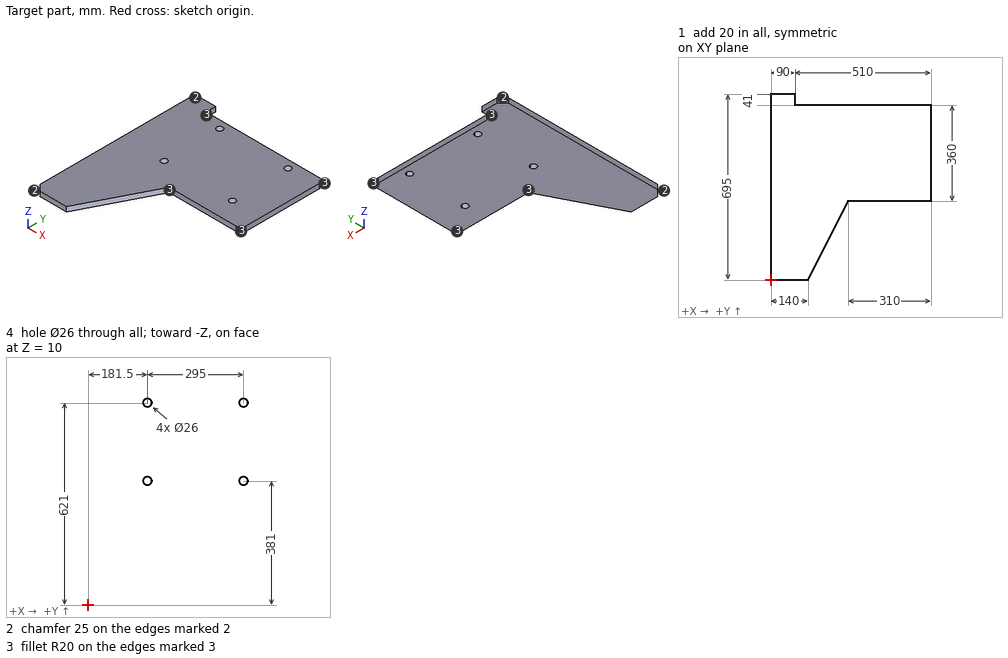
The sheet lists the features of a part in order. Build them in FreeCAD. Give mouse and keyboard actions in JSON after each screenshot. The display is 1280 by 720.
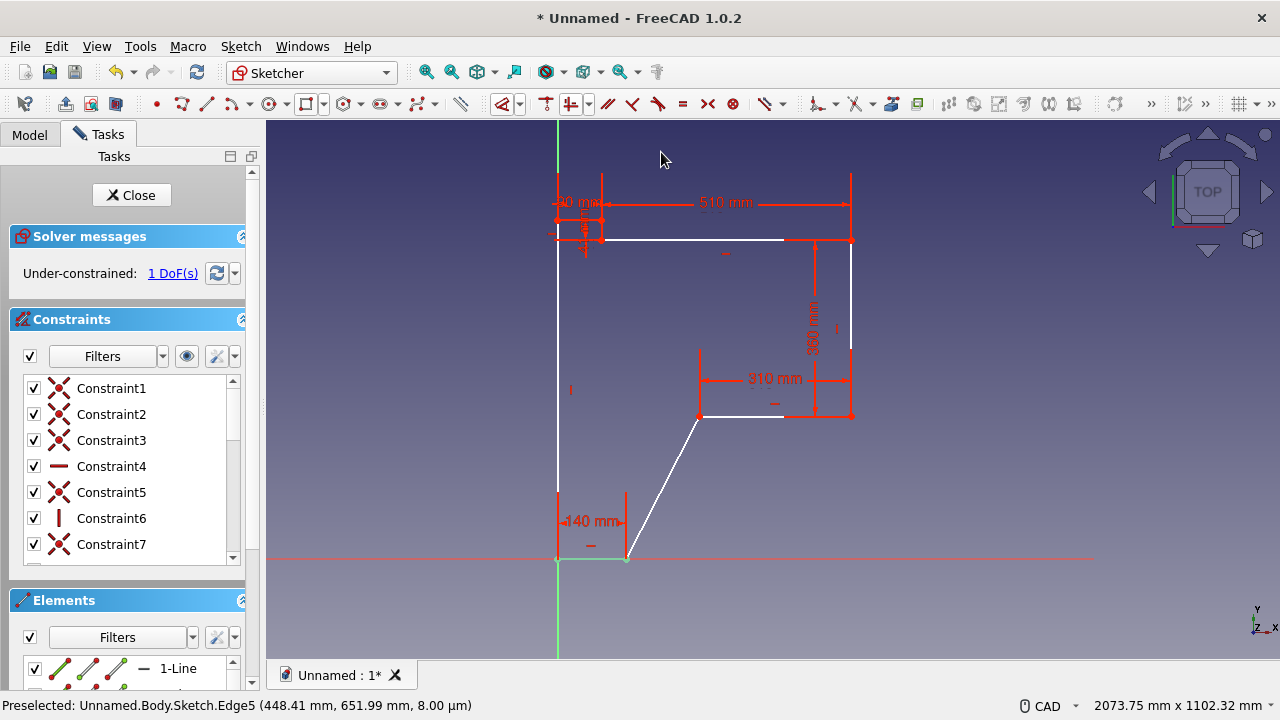
{"action": "left_click", "coordinate": [558, 322]}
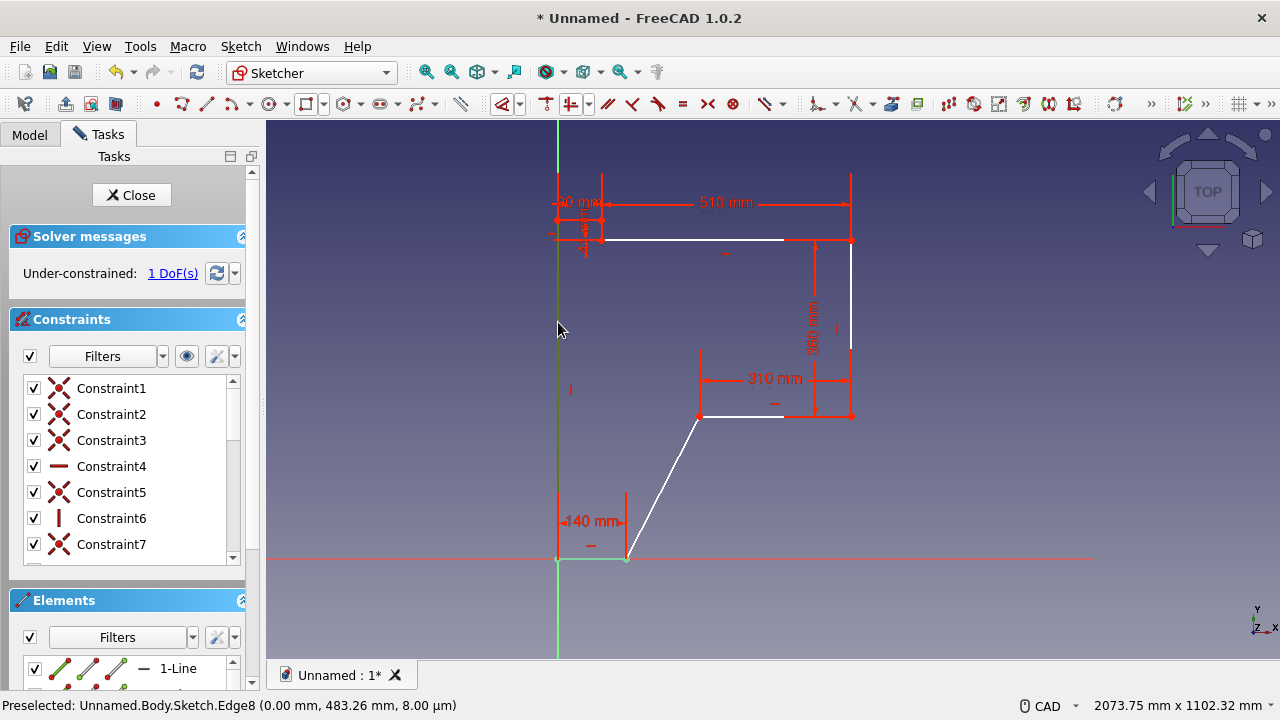
{"action": "left_click", "coordinate": [520, 104]}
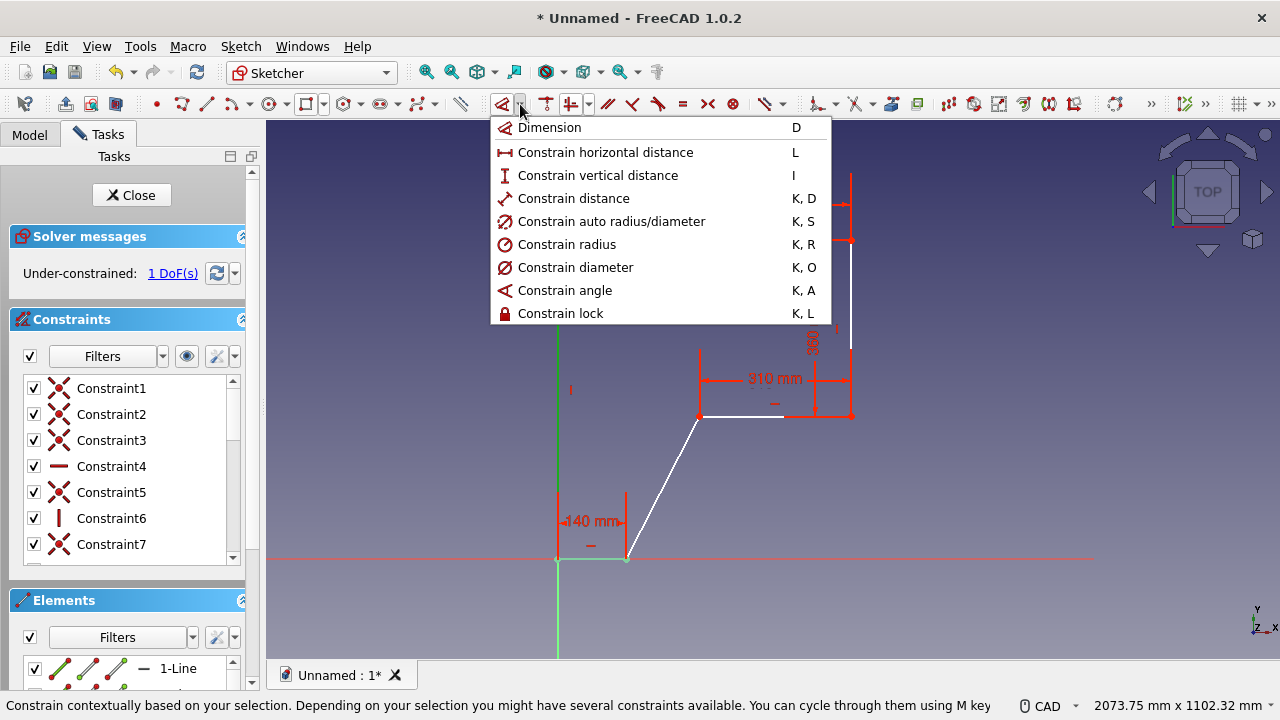
{"action": "left_click", "coordinate": [661, 176]}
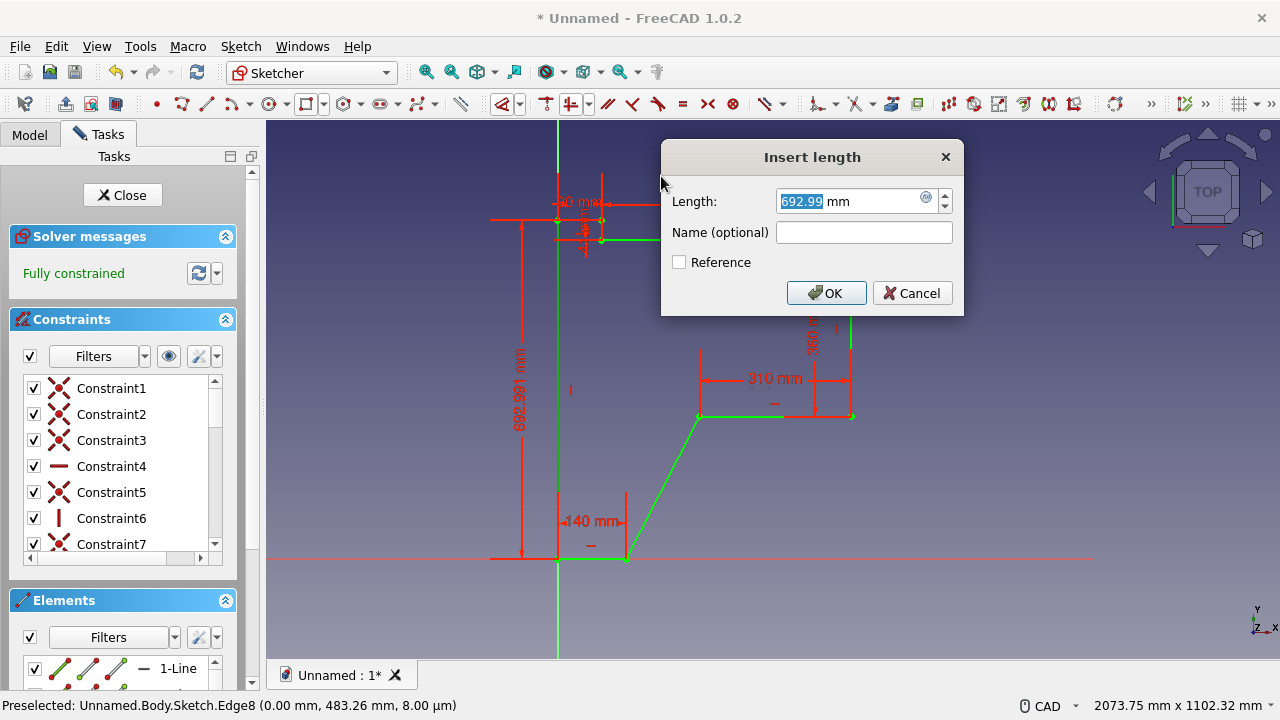
{"action": "type", "text": "695"}
{"action": "key", "text": "Return"}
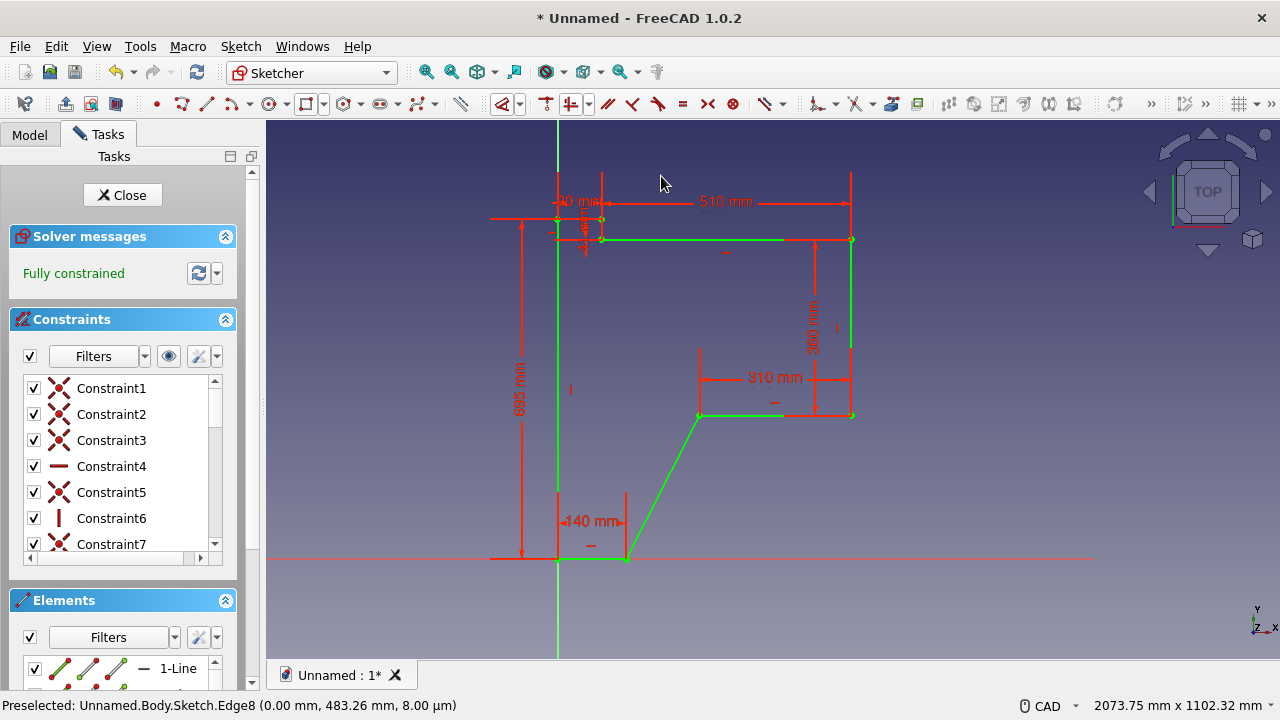
{"action": "left_click", "coordinate": [123, 195]}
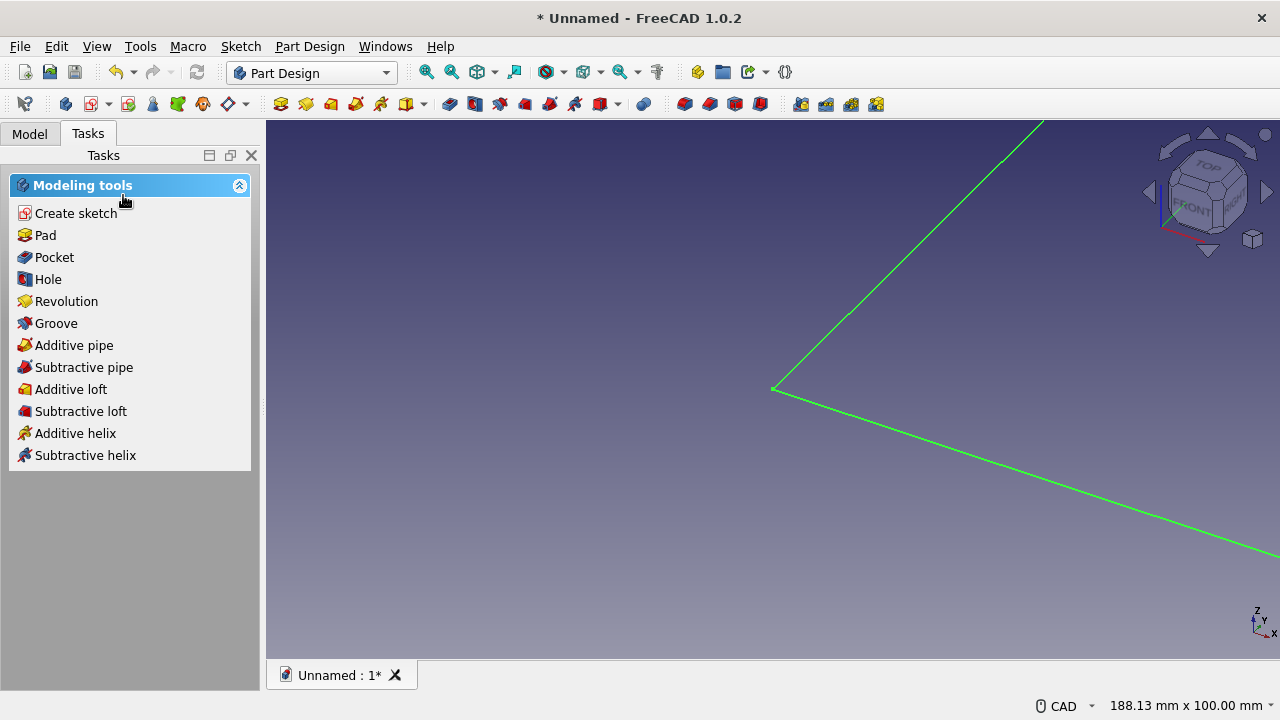
{"action": "left_click", "coordinate": [281, 104]}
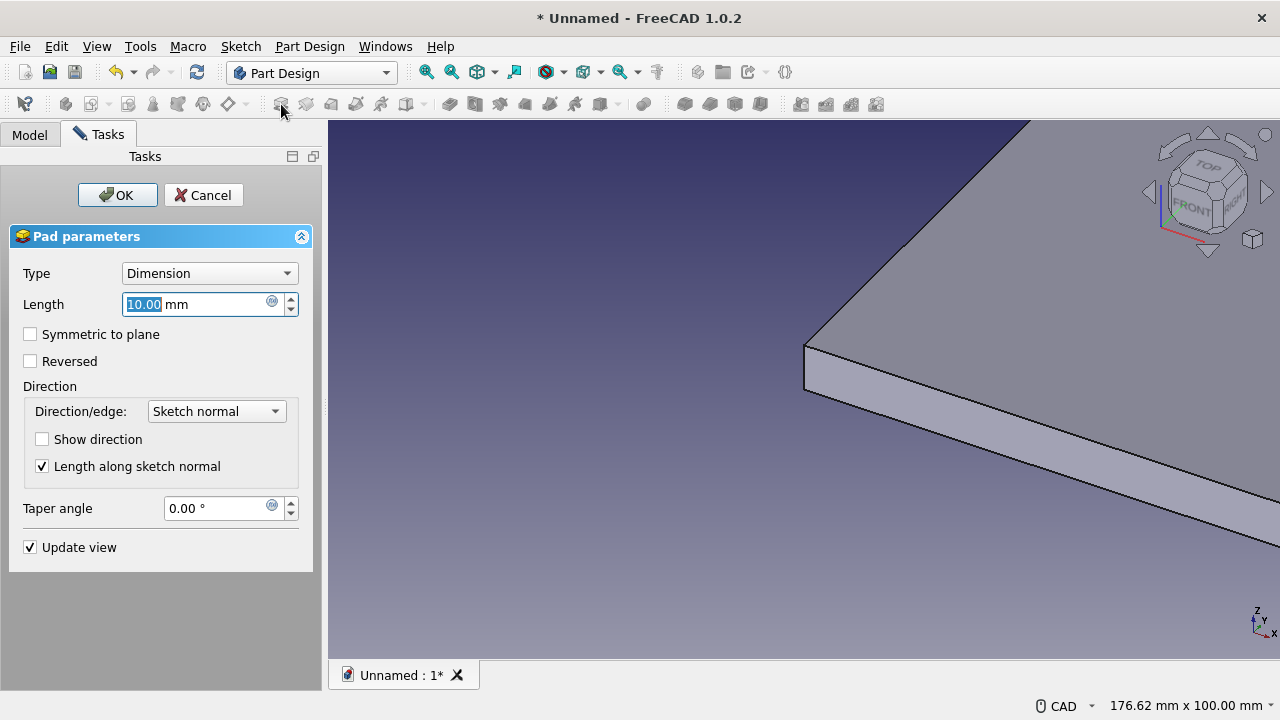
{"action": "type", "text": "20"}
{"action": "key", "text": "Tab"}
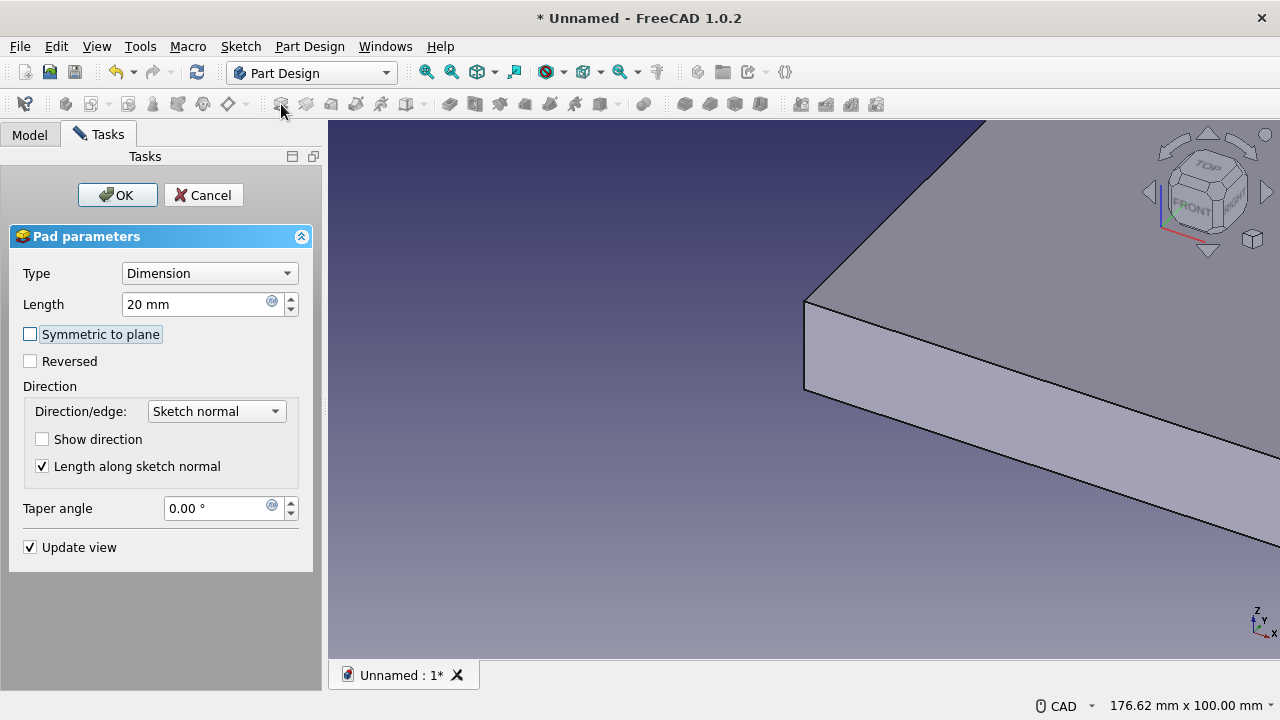
{"action": "left_click", "coordinate": [31, 334]}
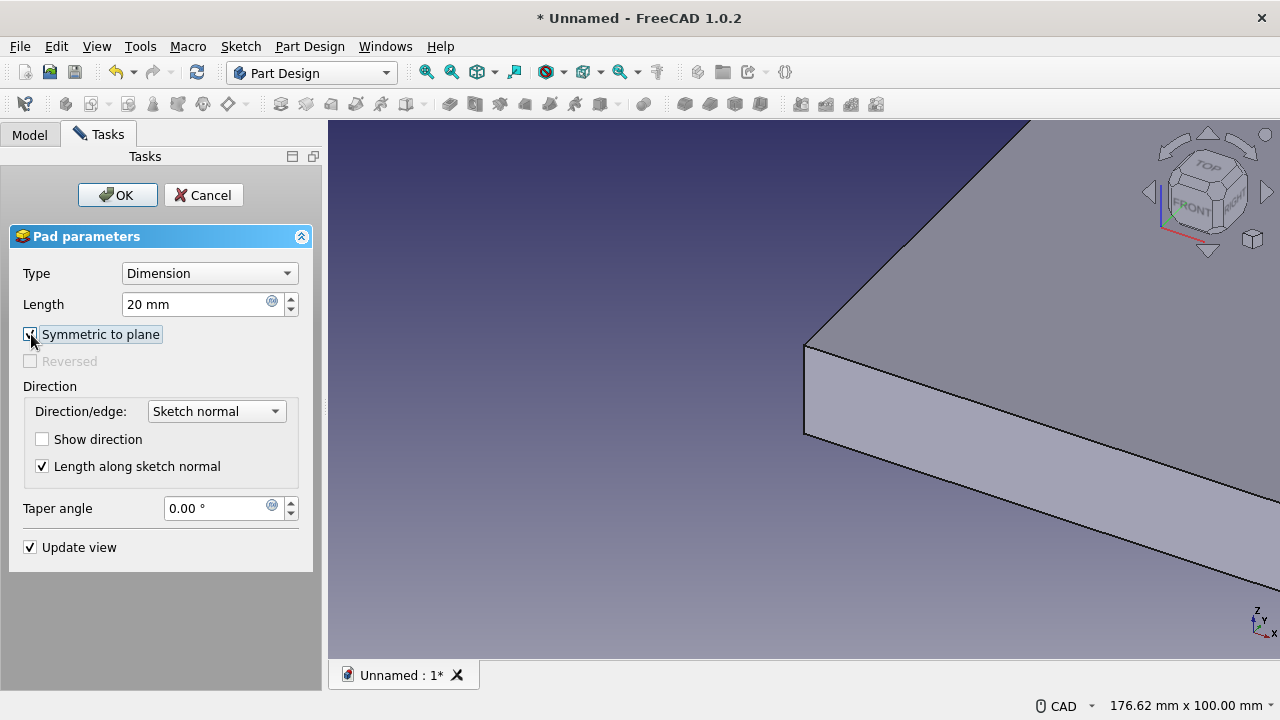
{"action": "left_click", "coordinate": [118, 195]}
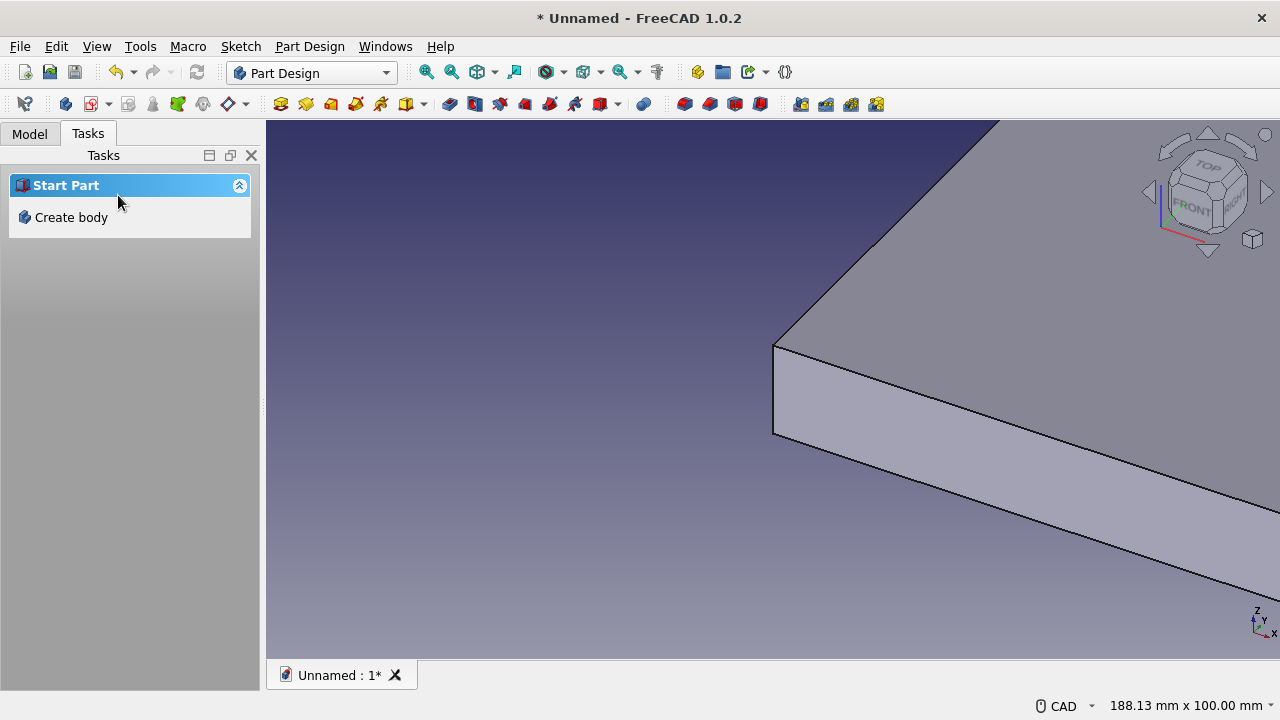
{"action": "left_click", "coordinate": [427, 72]}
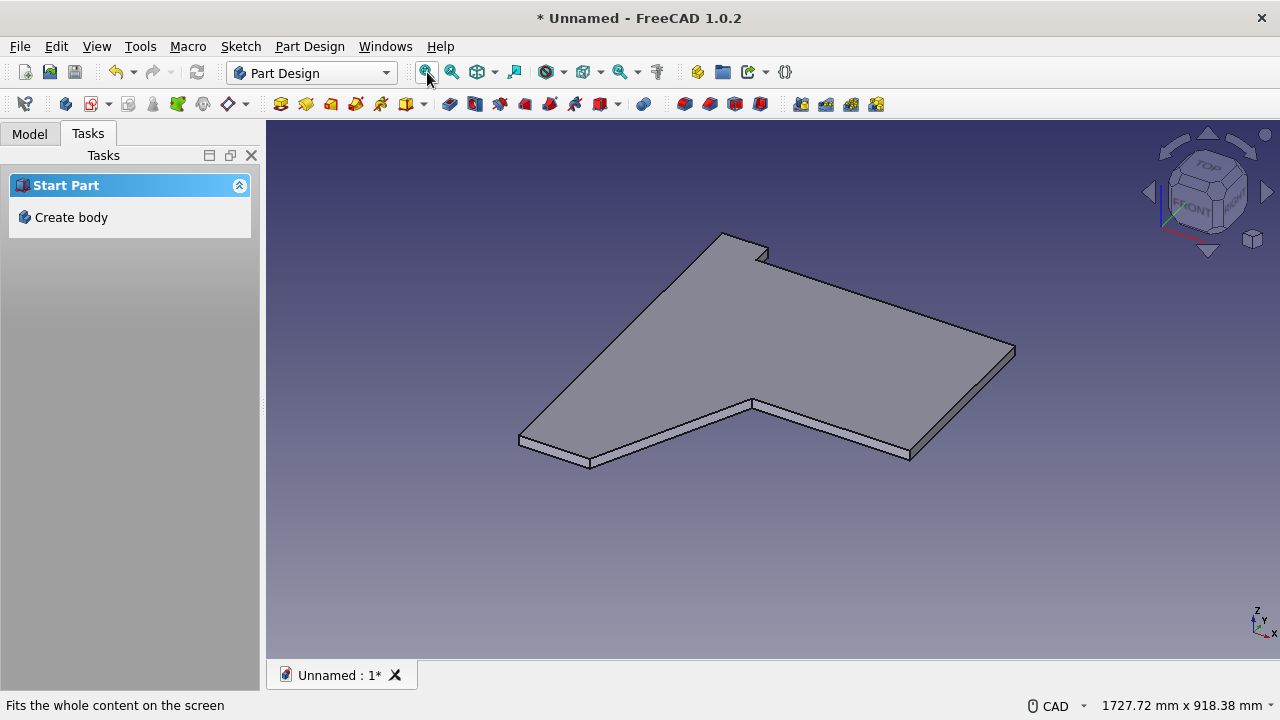
{"action": "scroll", "coordinate": [519, 439], "scroll_direction": "up", "scroll_amount": 7}